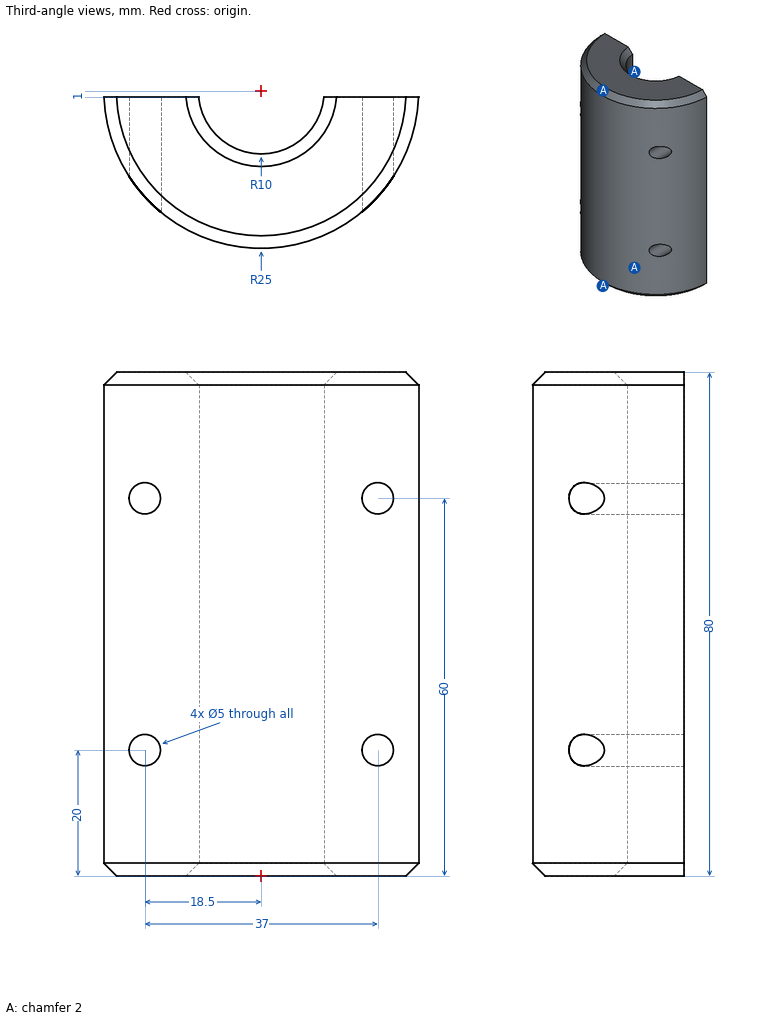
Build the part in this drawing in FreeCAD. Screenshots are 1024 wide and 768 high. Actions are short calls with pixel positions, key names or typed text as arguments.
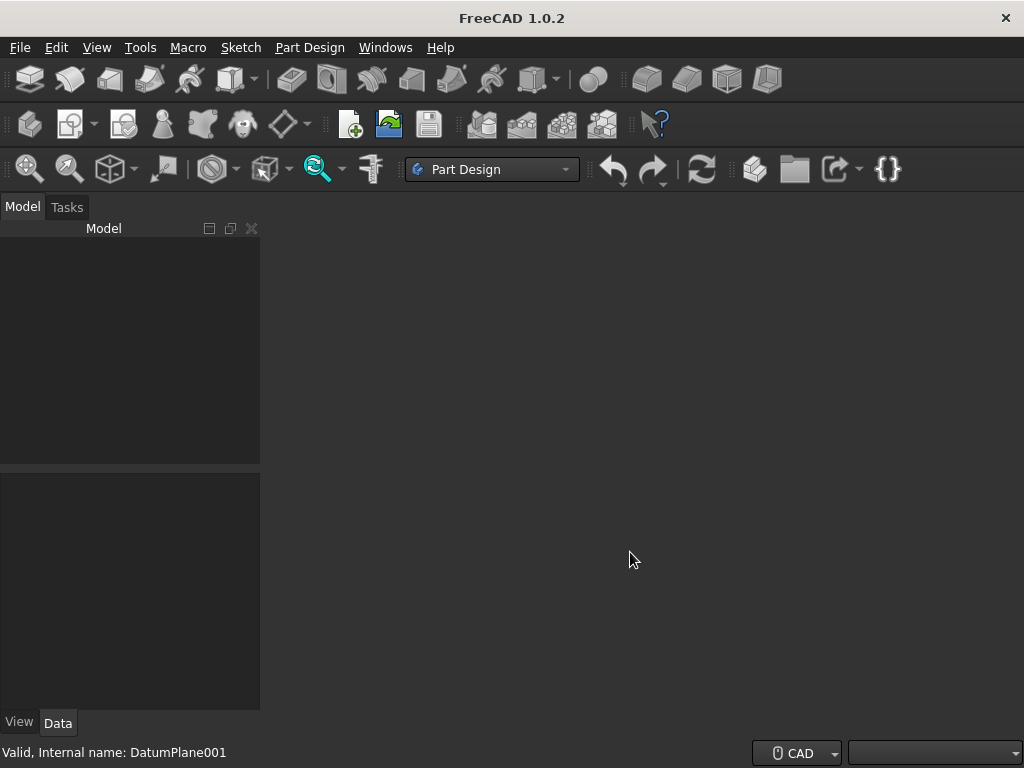
click(350, 124)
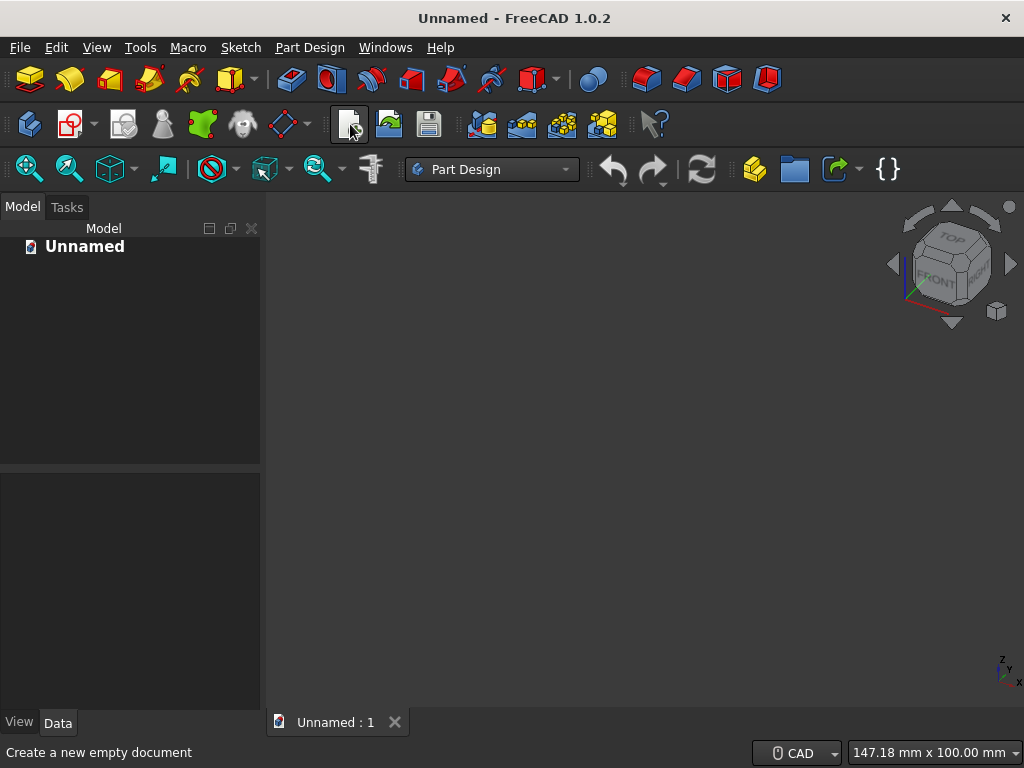
click(70, 124)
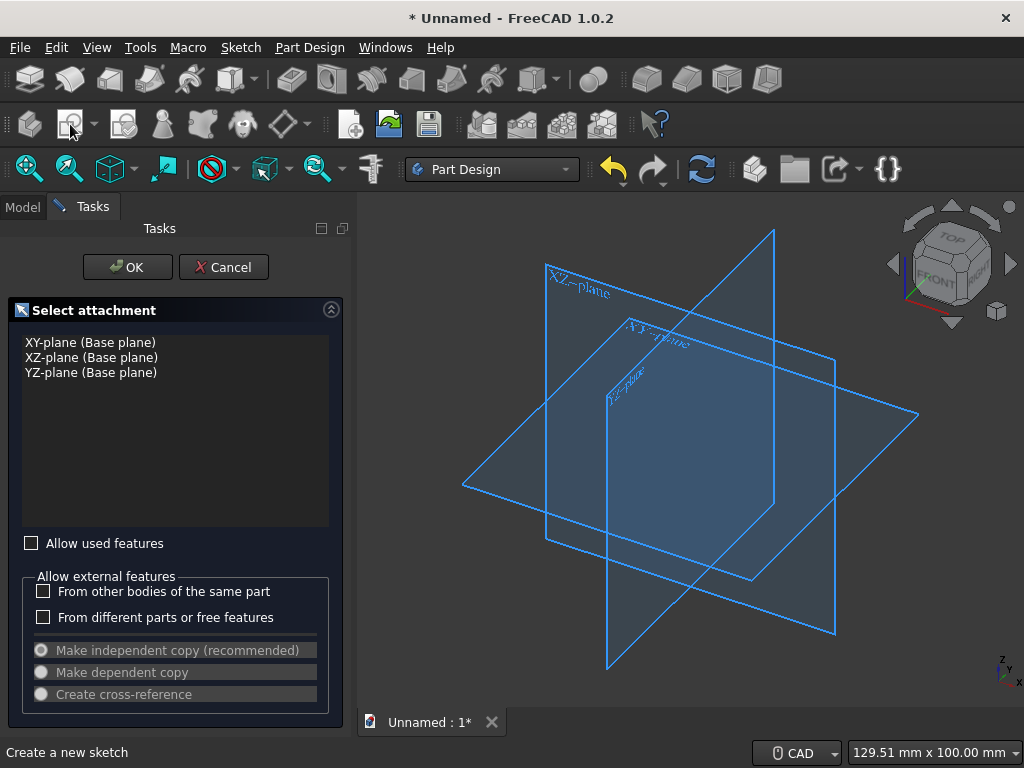
click(82, 342)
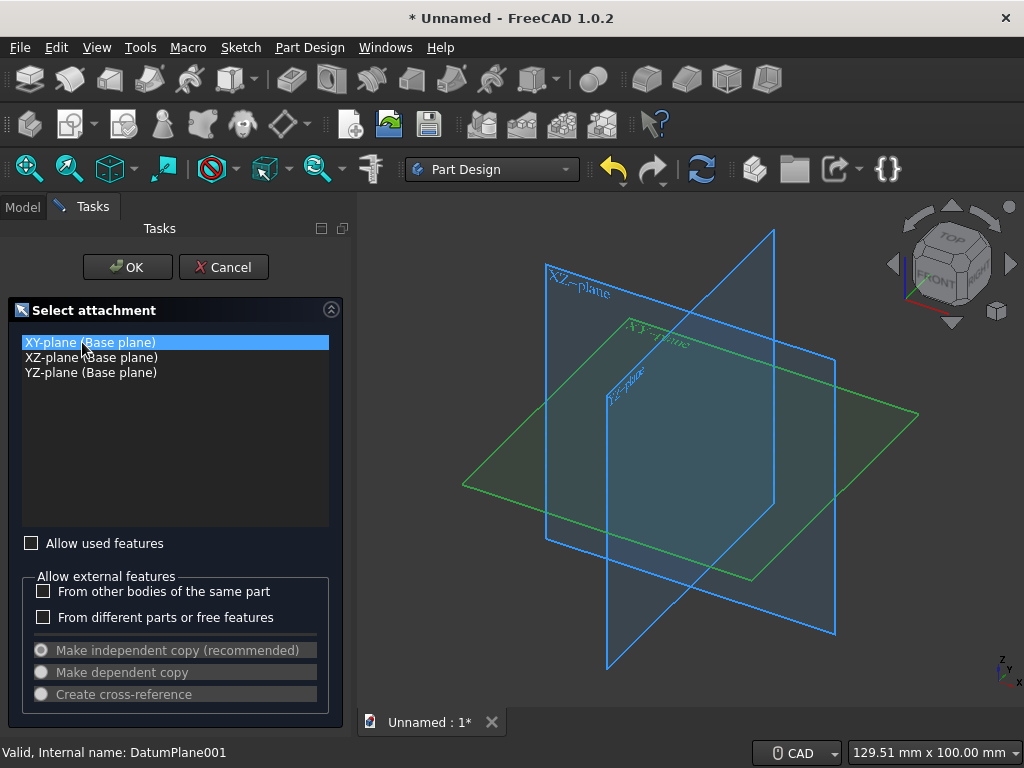
click(128, 267)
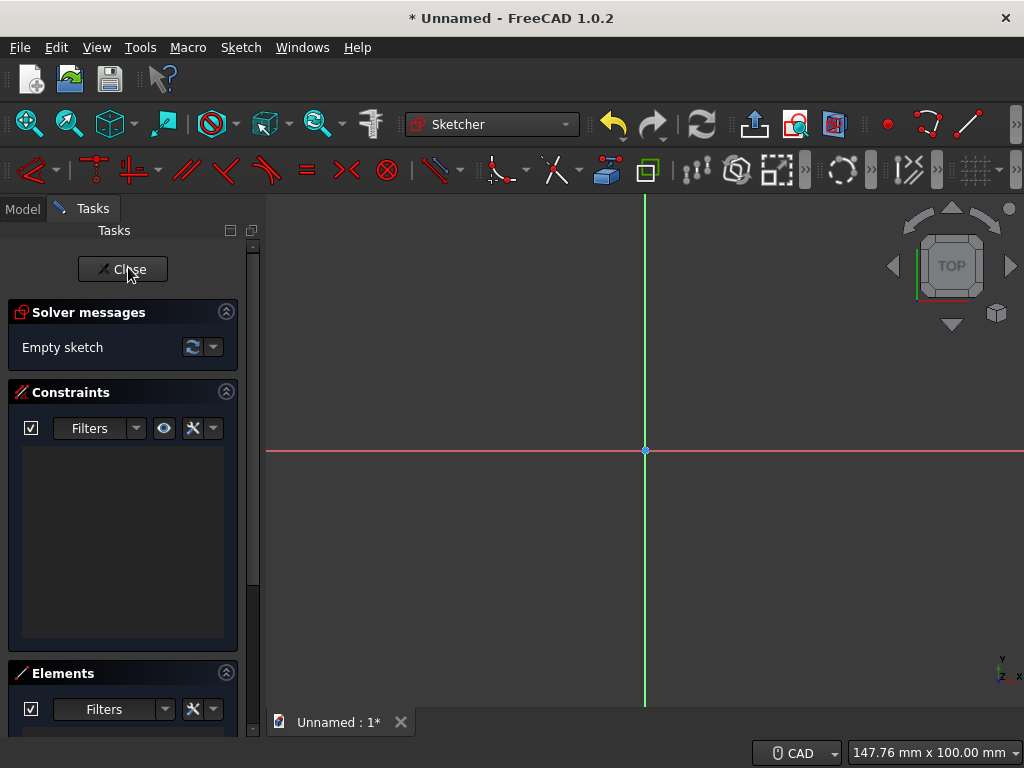
scroll(784, 645, up, 2)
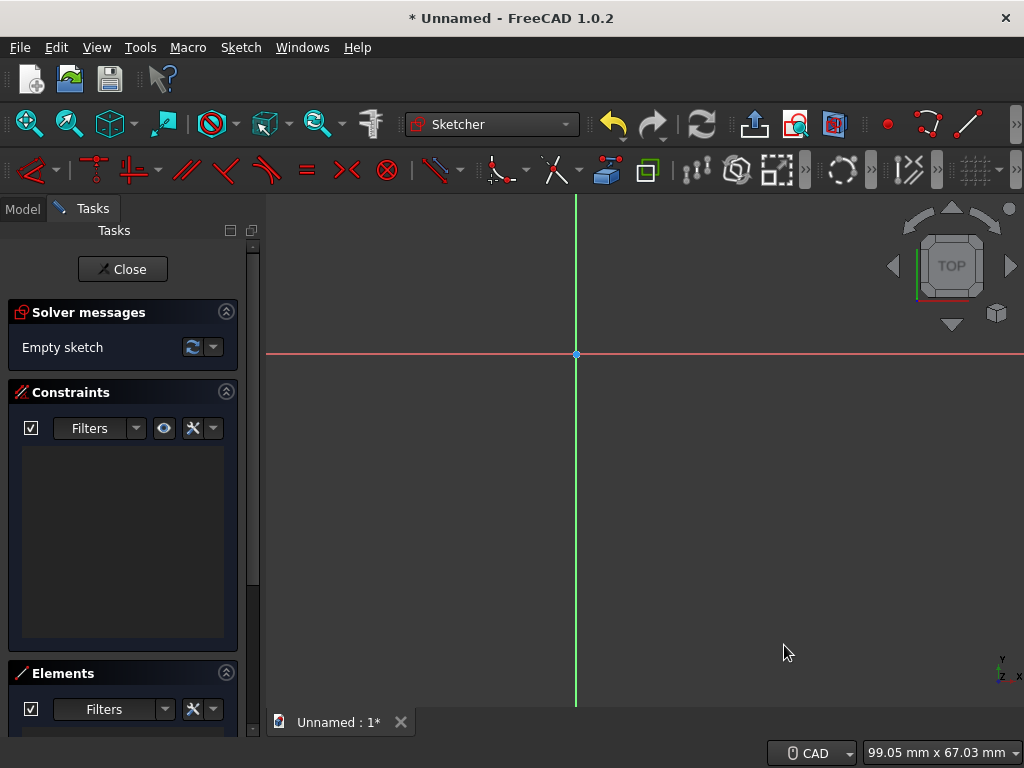
click(968, 124)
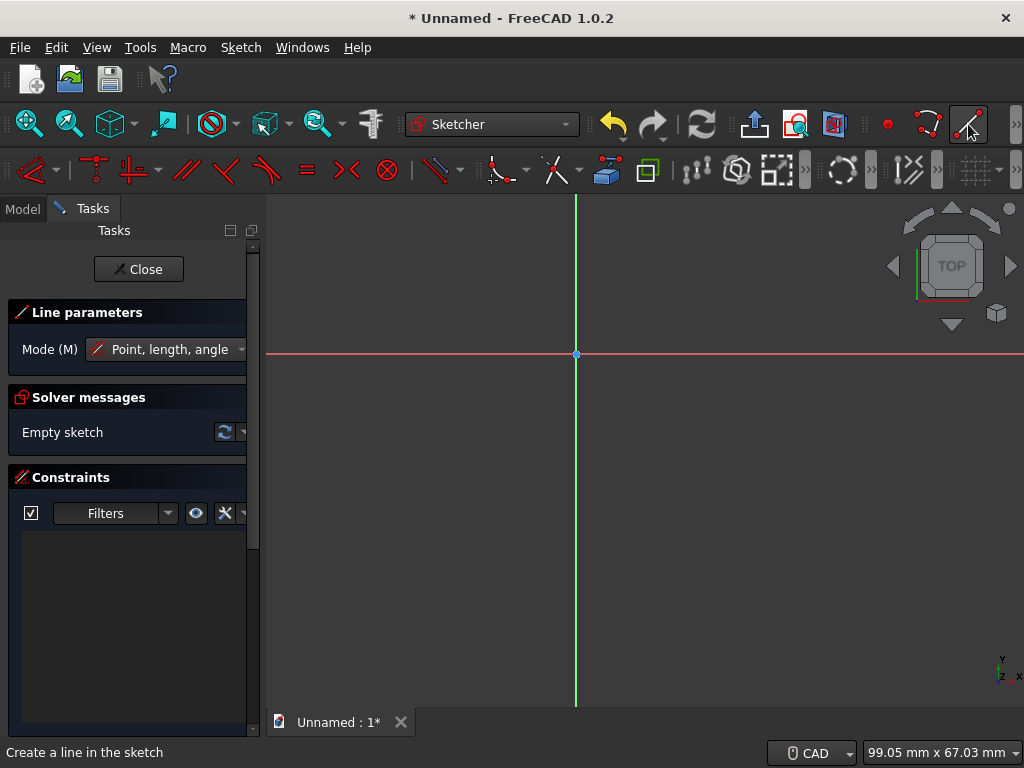
scroll(500, 362, up, 4)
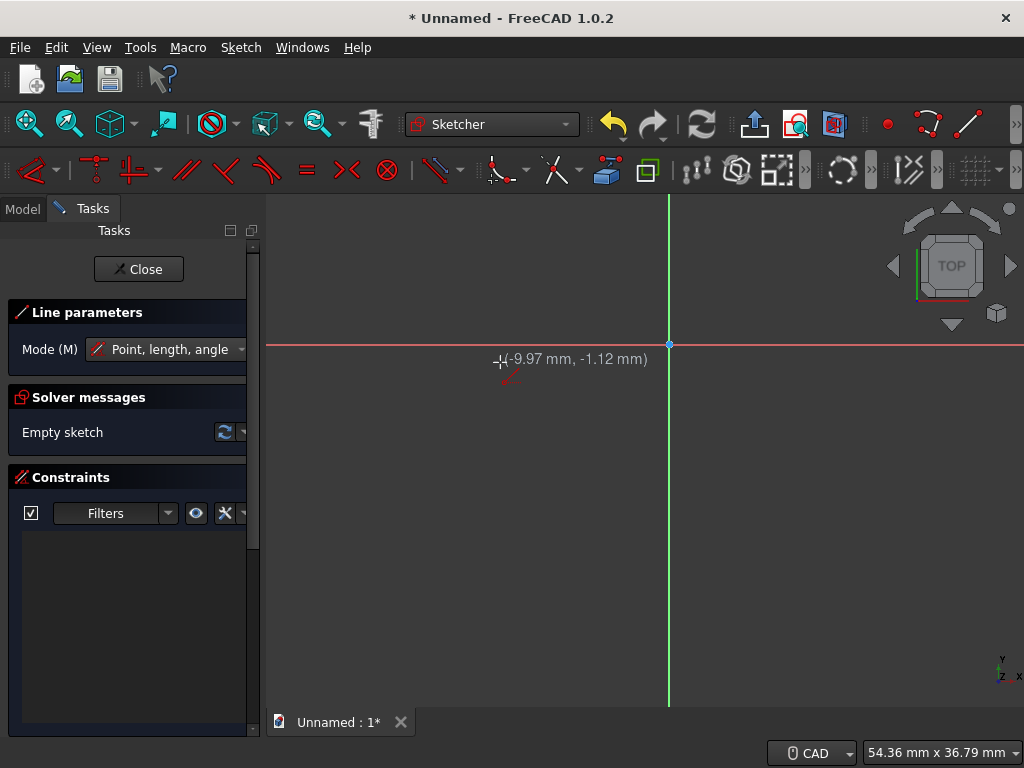
click(500, 362)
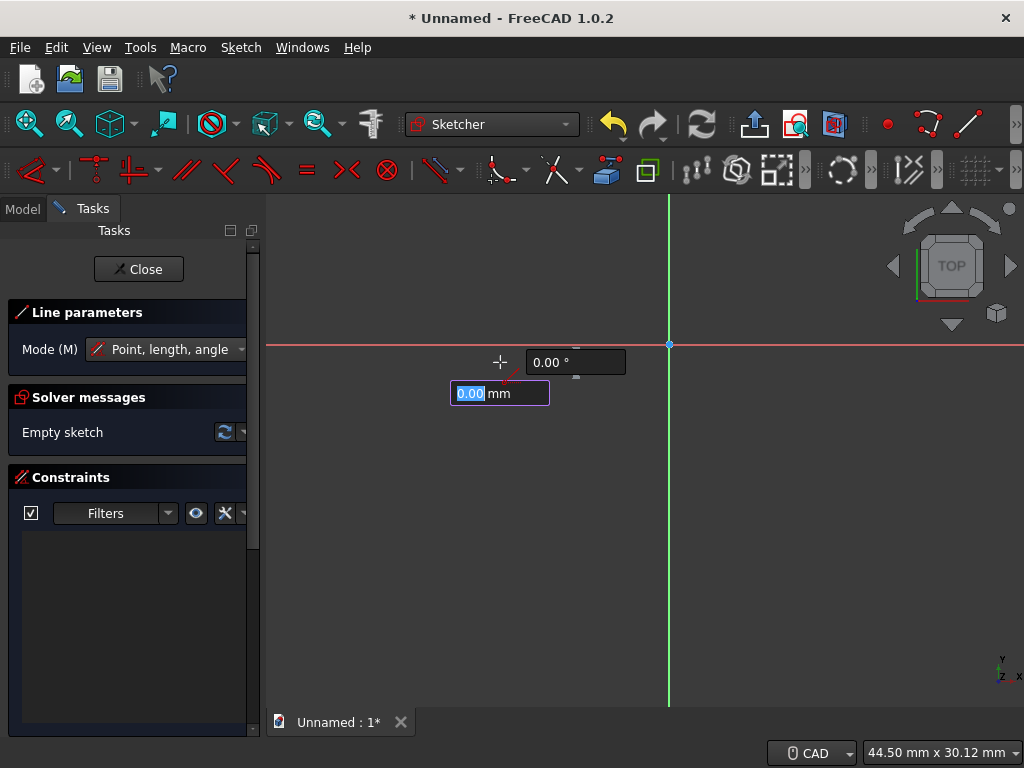
scroll(501, 363, down, 4)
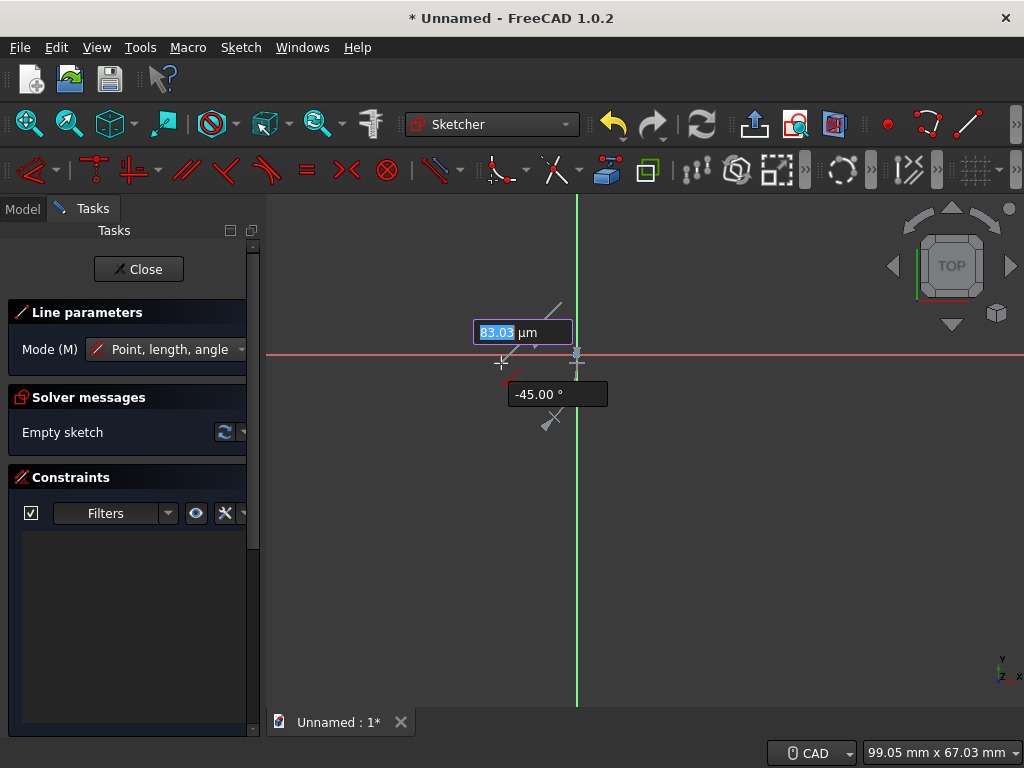
scroll(386, 363, up, 4)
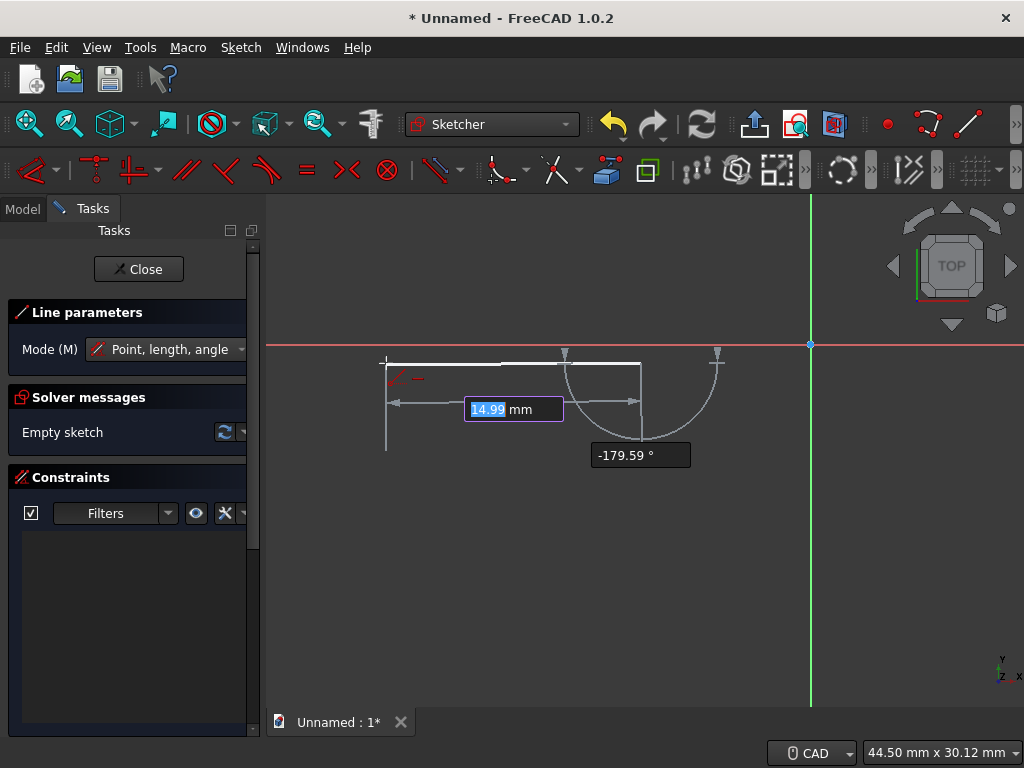
click(385, 362)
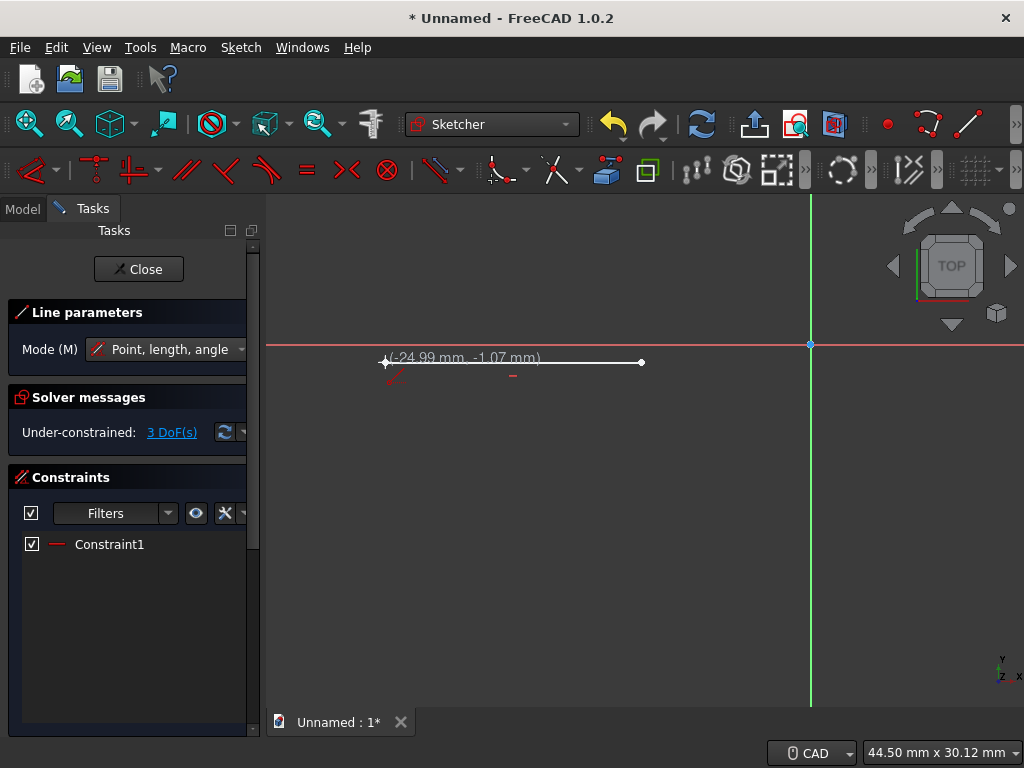
scroll(386, 363, down, 4)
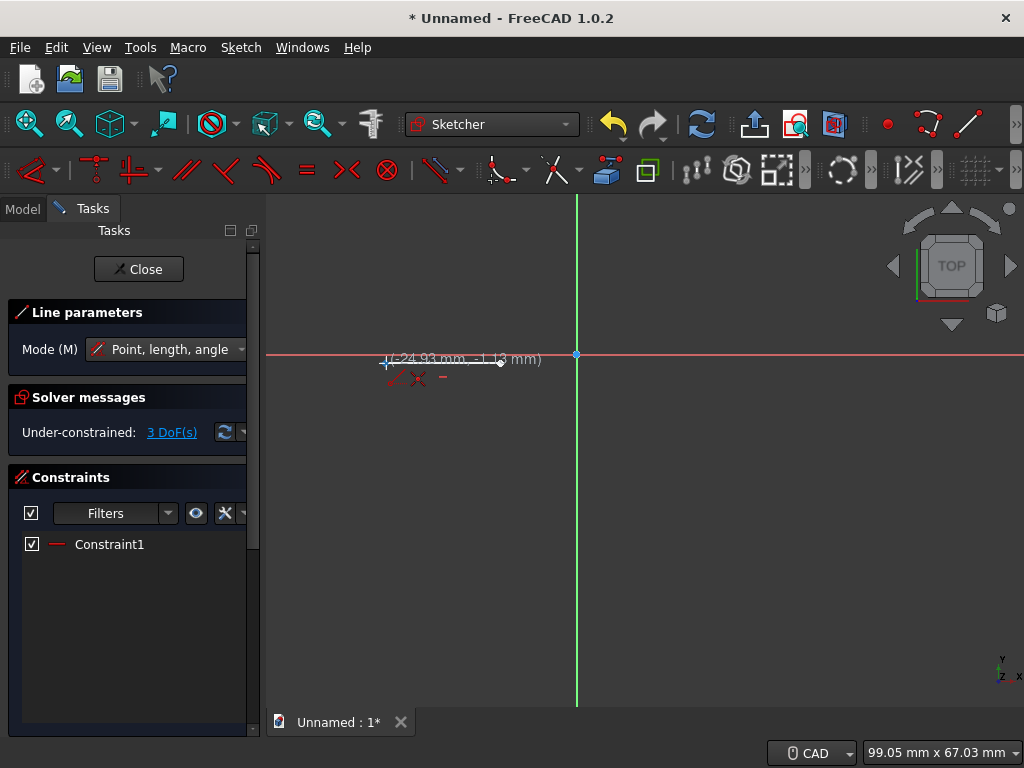
scroll(768, 363, up, 4)